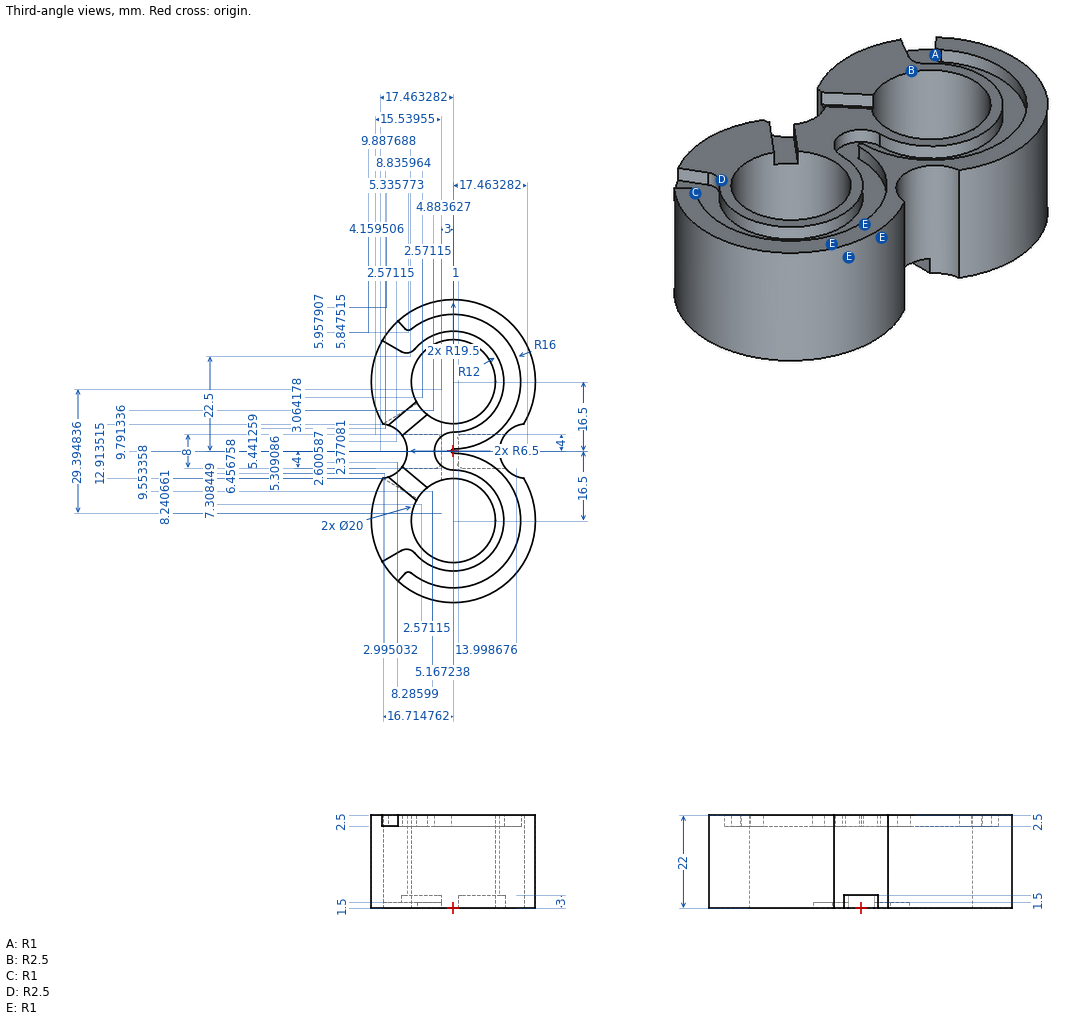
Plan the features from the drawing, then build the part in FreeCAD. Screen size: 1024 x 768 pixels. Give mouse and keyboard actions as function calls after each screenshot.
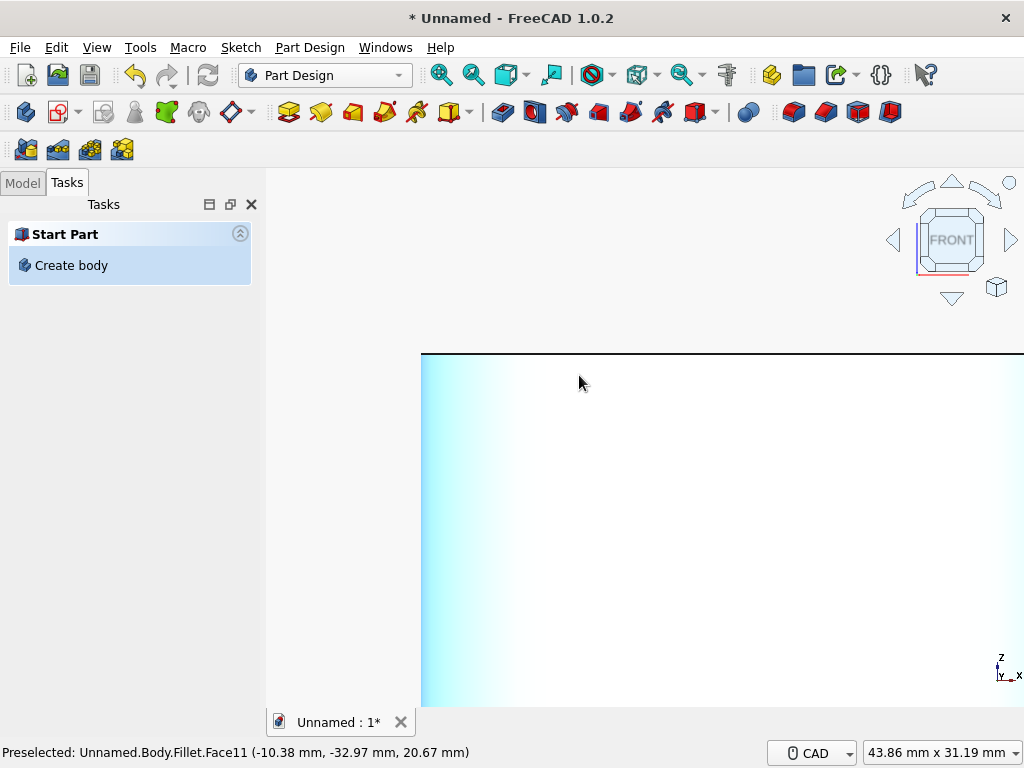
click(442, 76)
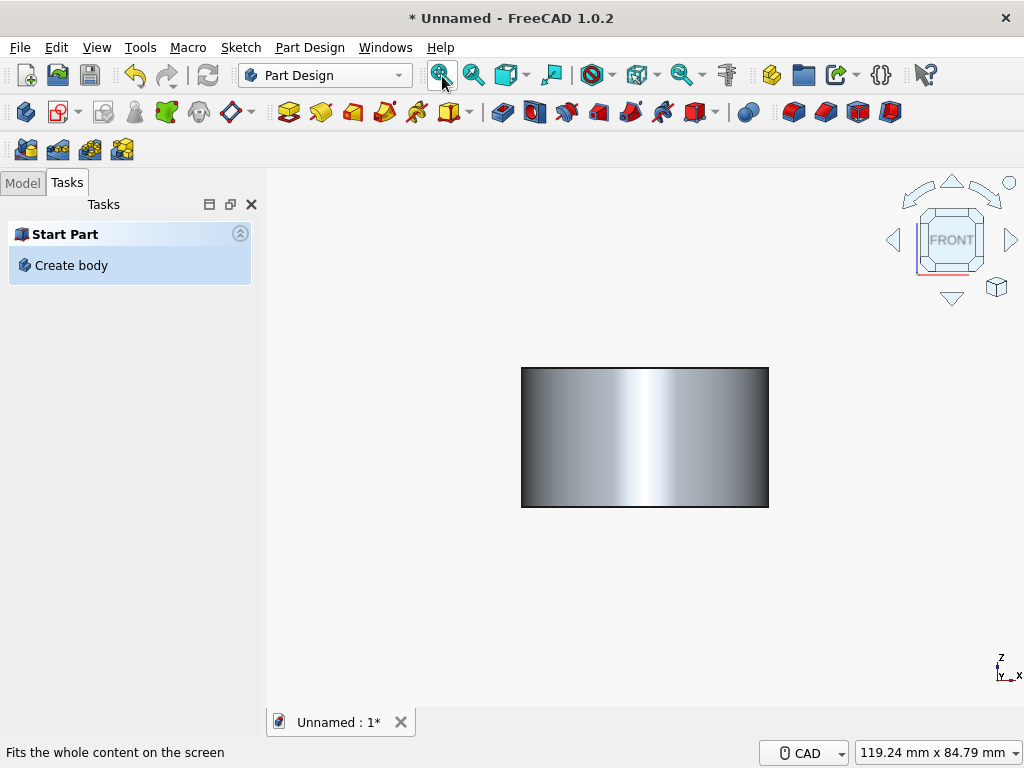
key(3)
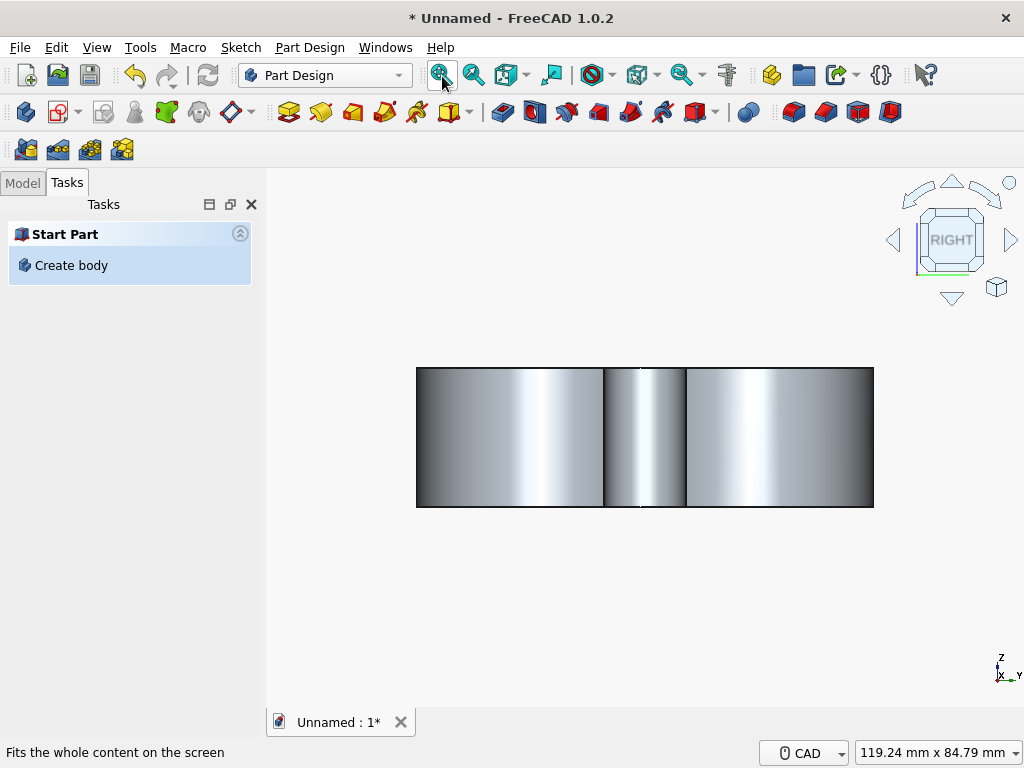
scroll(788, 375, up, 5)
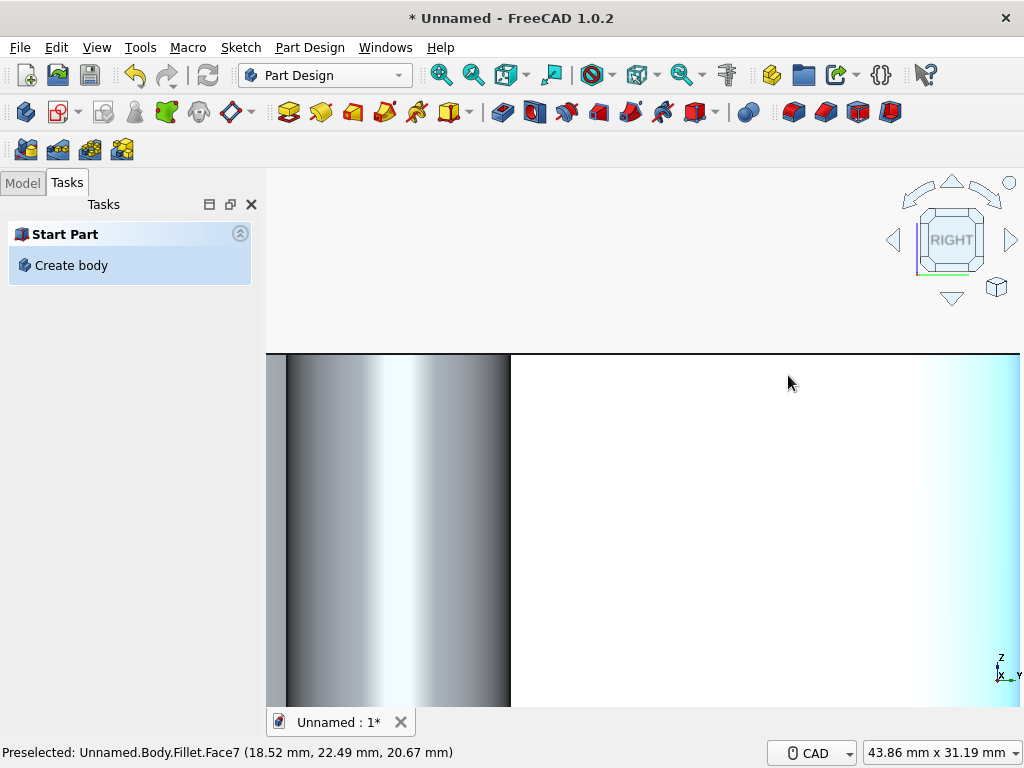
key(v)
key(f)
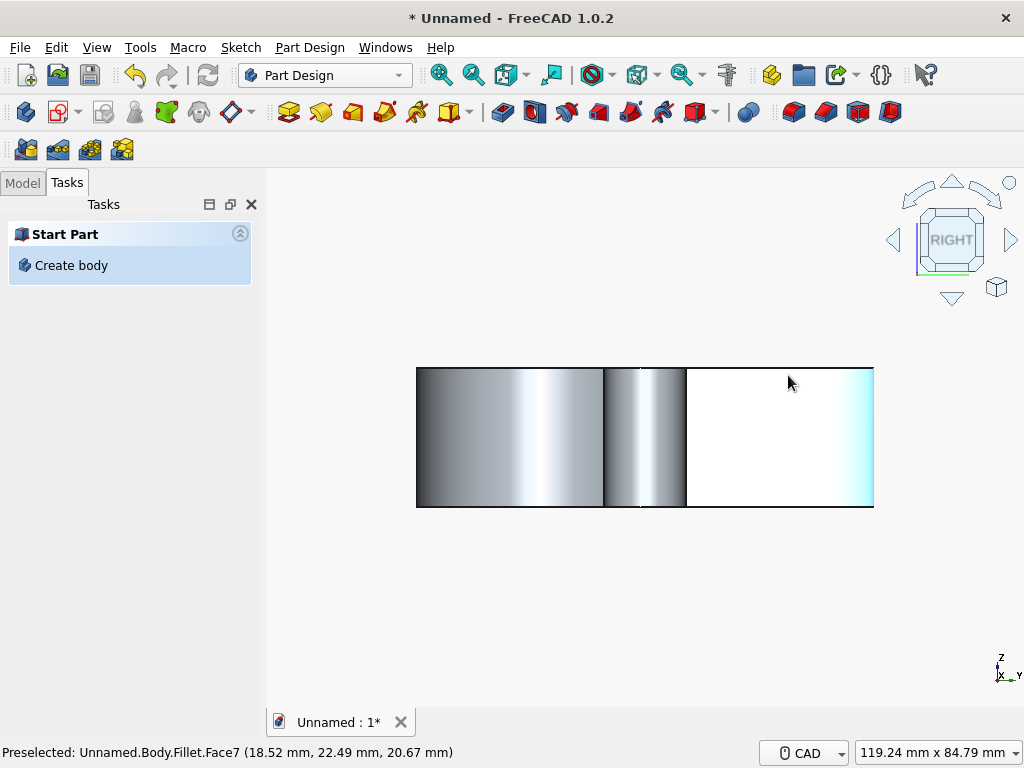
key(5)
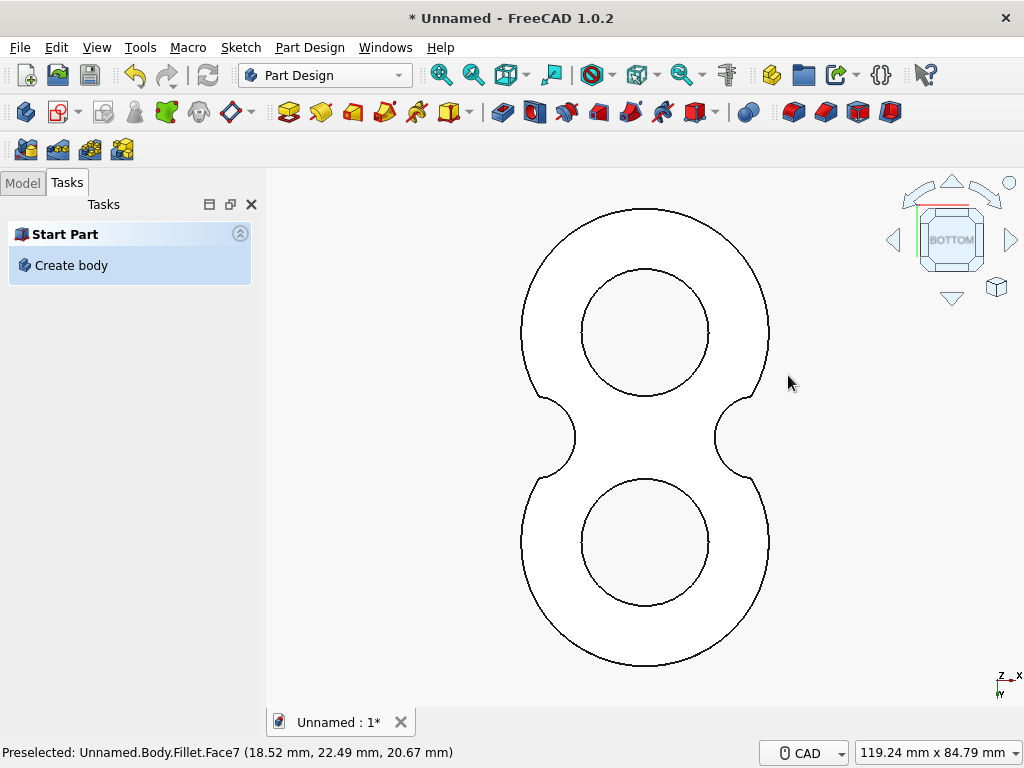
scroll(579, 580, up, 5)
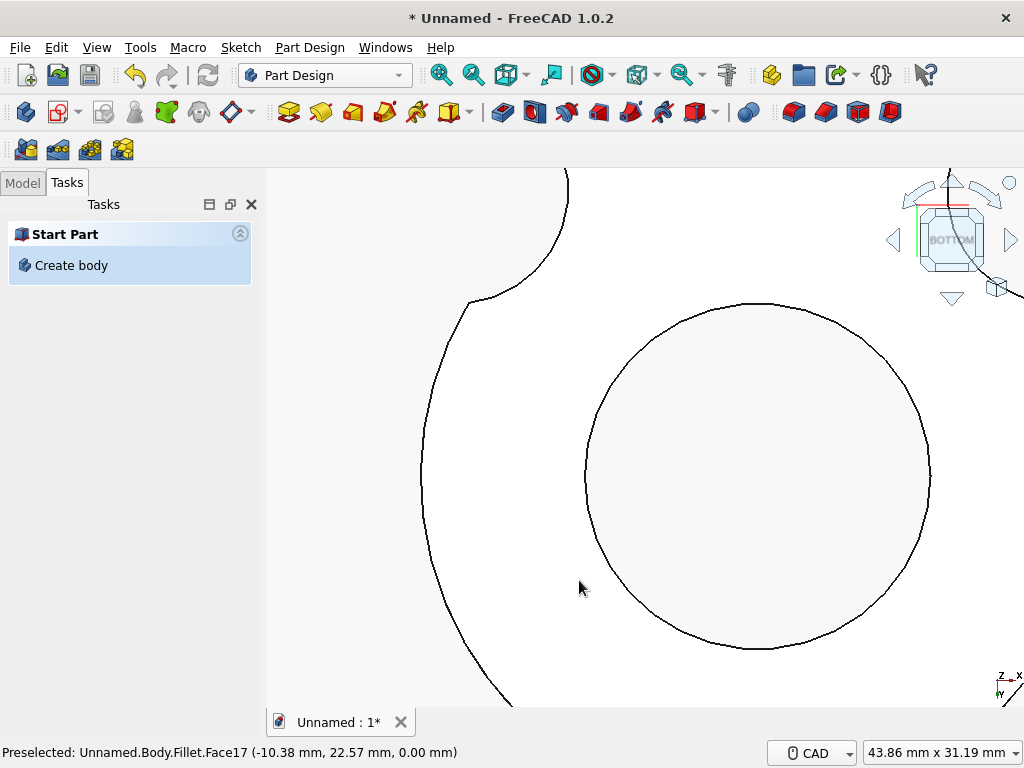
key(v)
key(f)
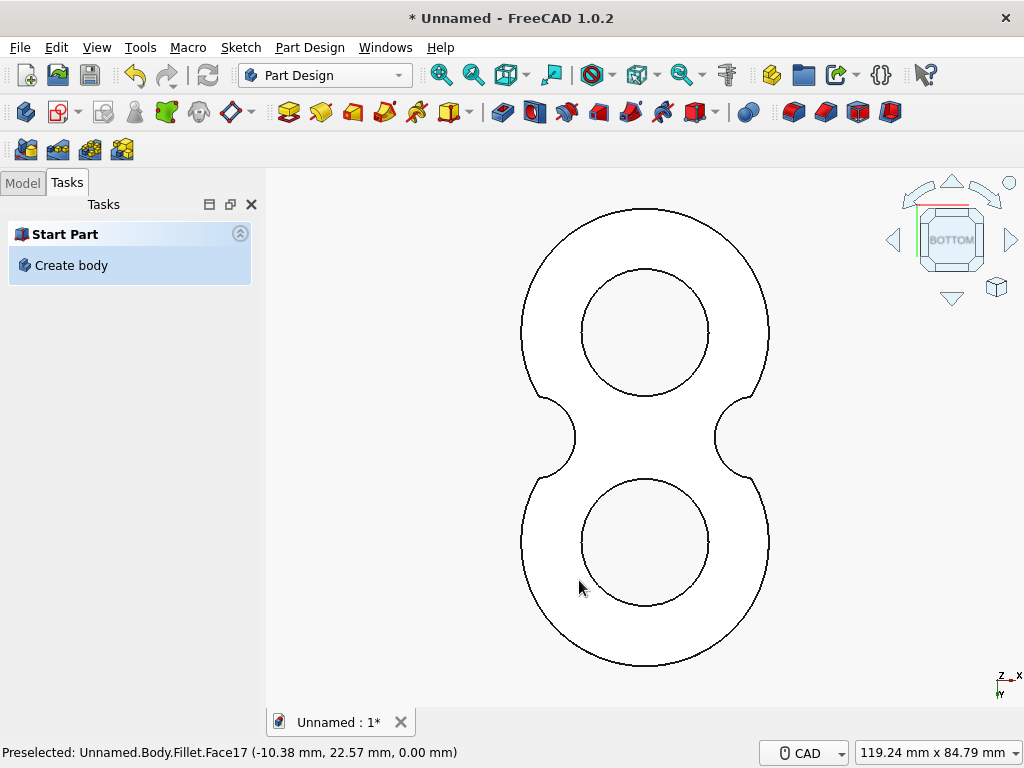
key(4)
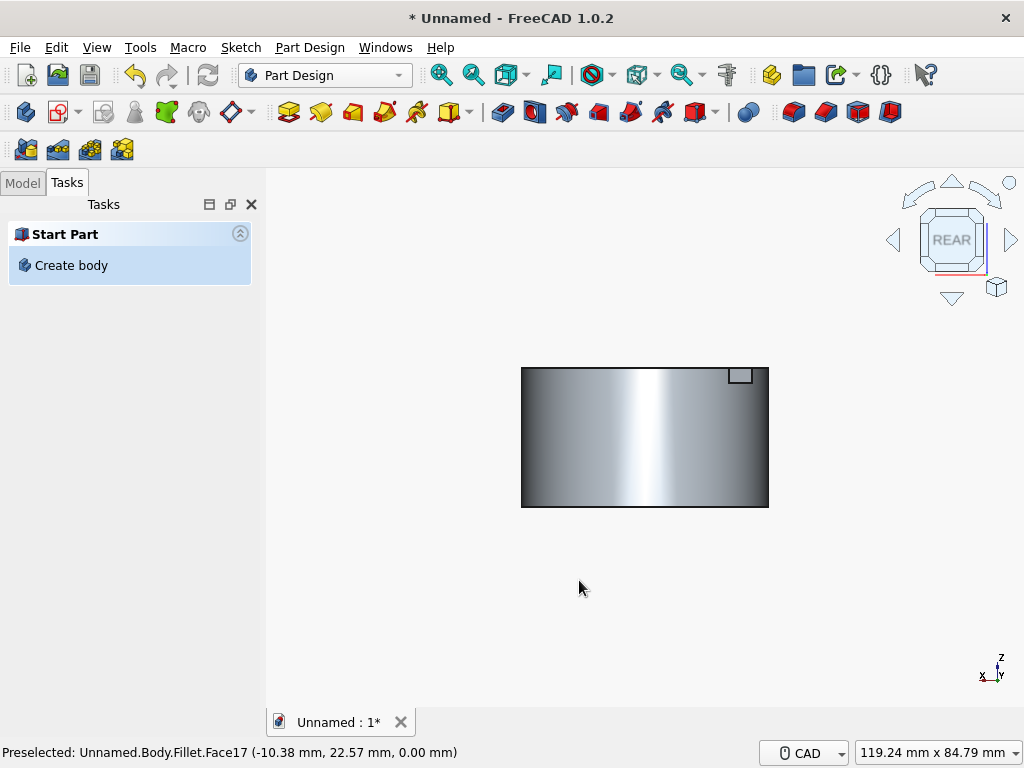
key(v)
key(f)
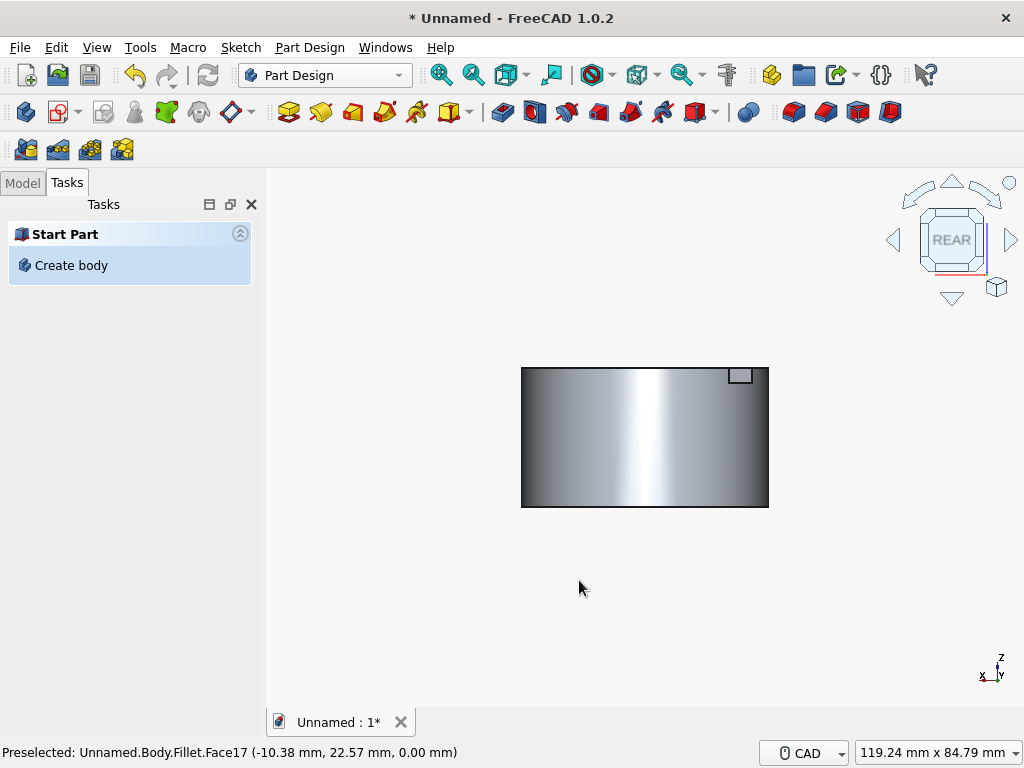
scroll(711, 375, up, 5)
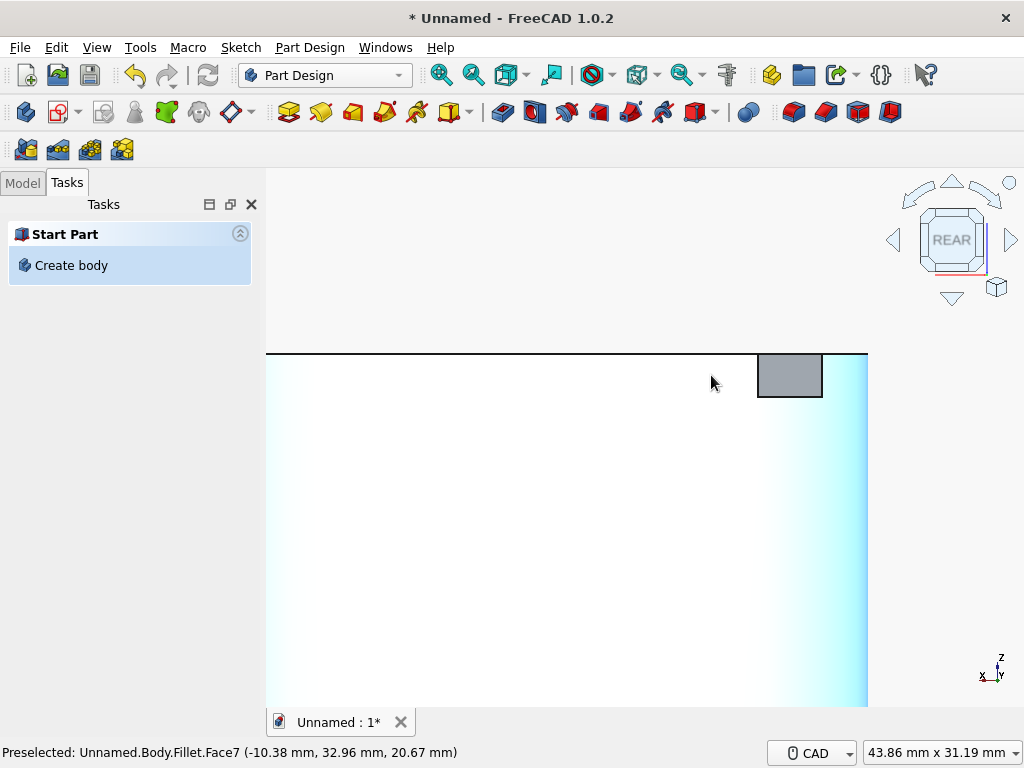
key(v)
key(f)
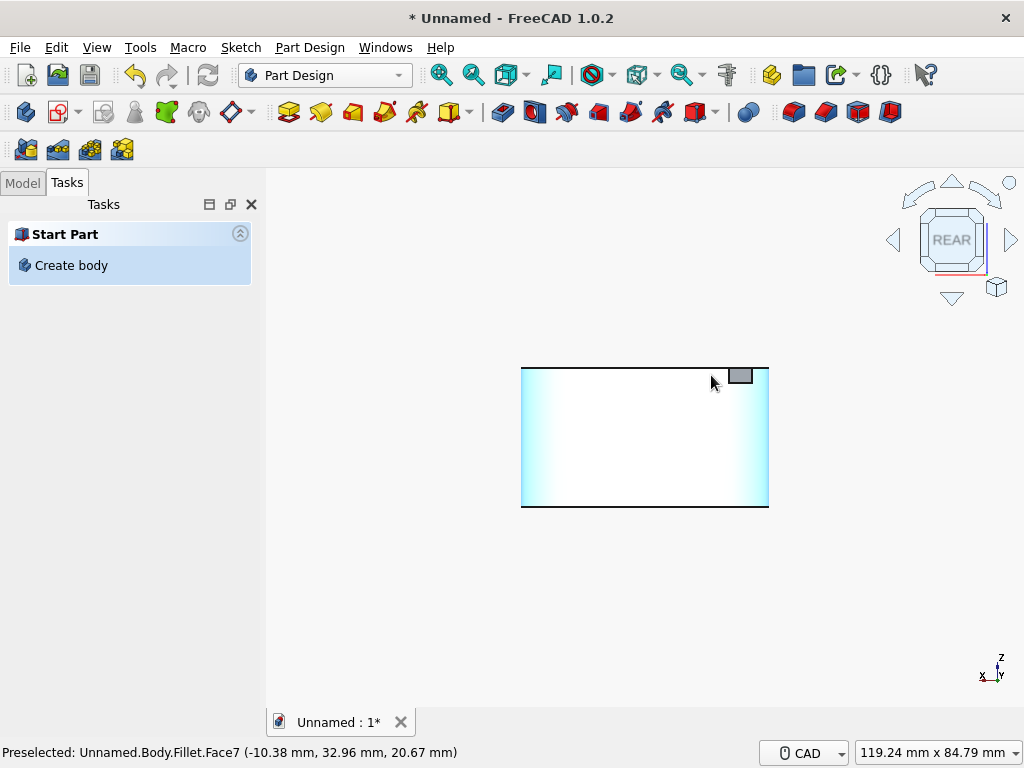
key(6)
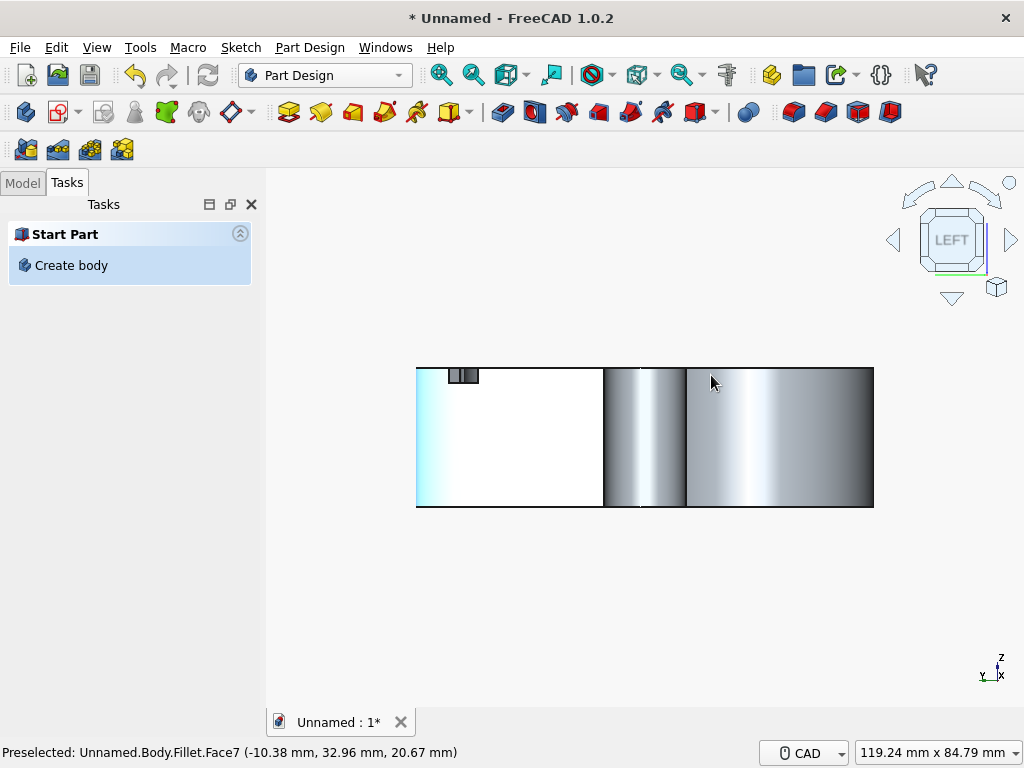
scroll(502, 375, up, 5)